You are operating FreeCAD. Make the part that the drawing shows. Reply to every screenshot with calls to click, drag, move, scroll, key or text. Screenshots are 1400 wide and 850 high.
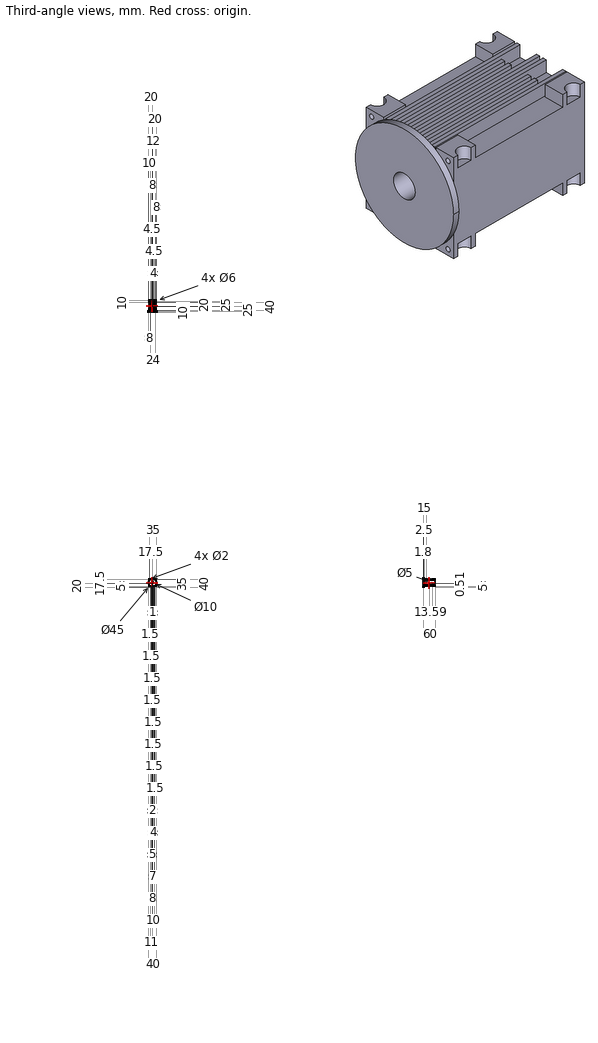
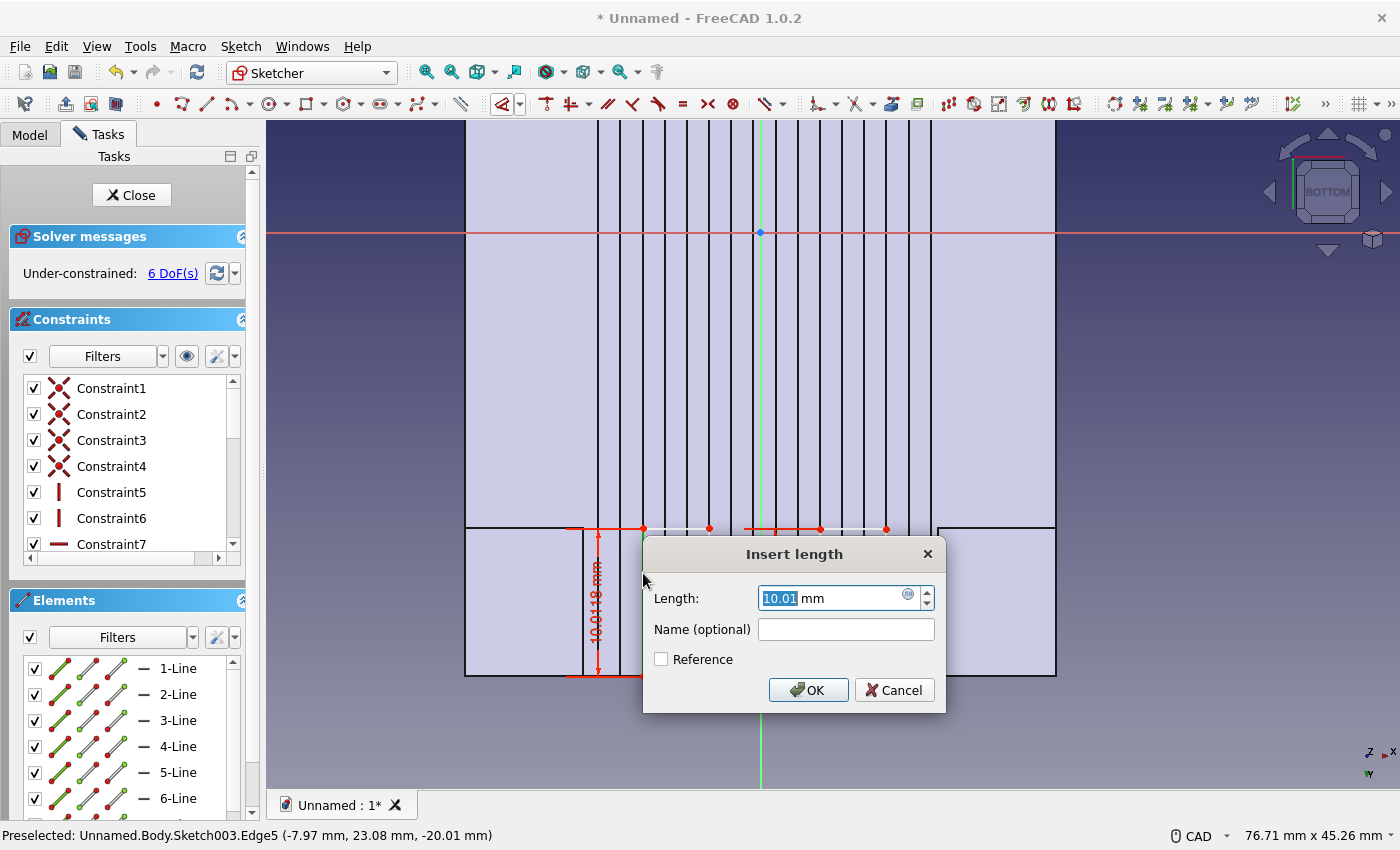
text(10)
key(Return)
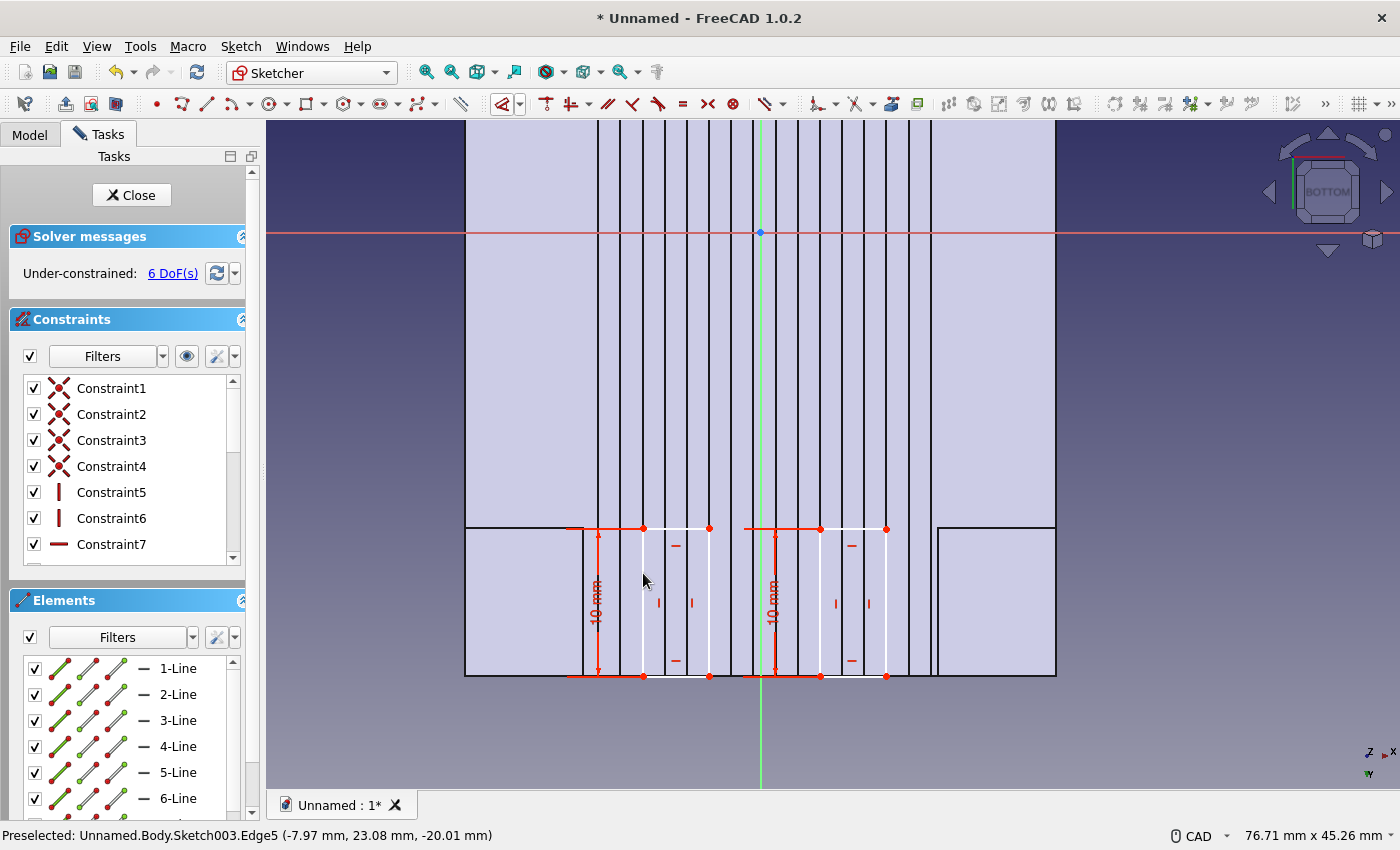
click(820, 529)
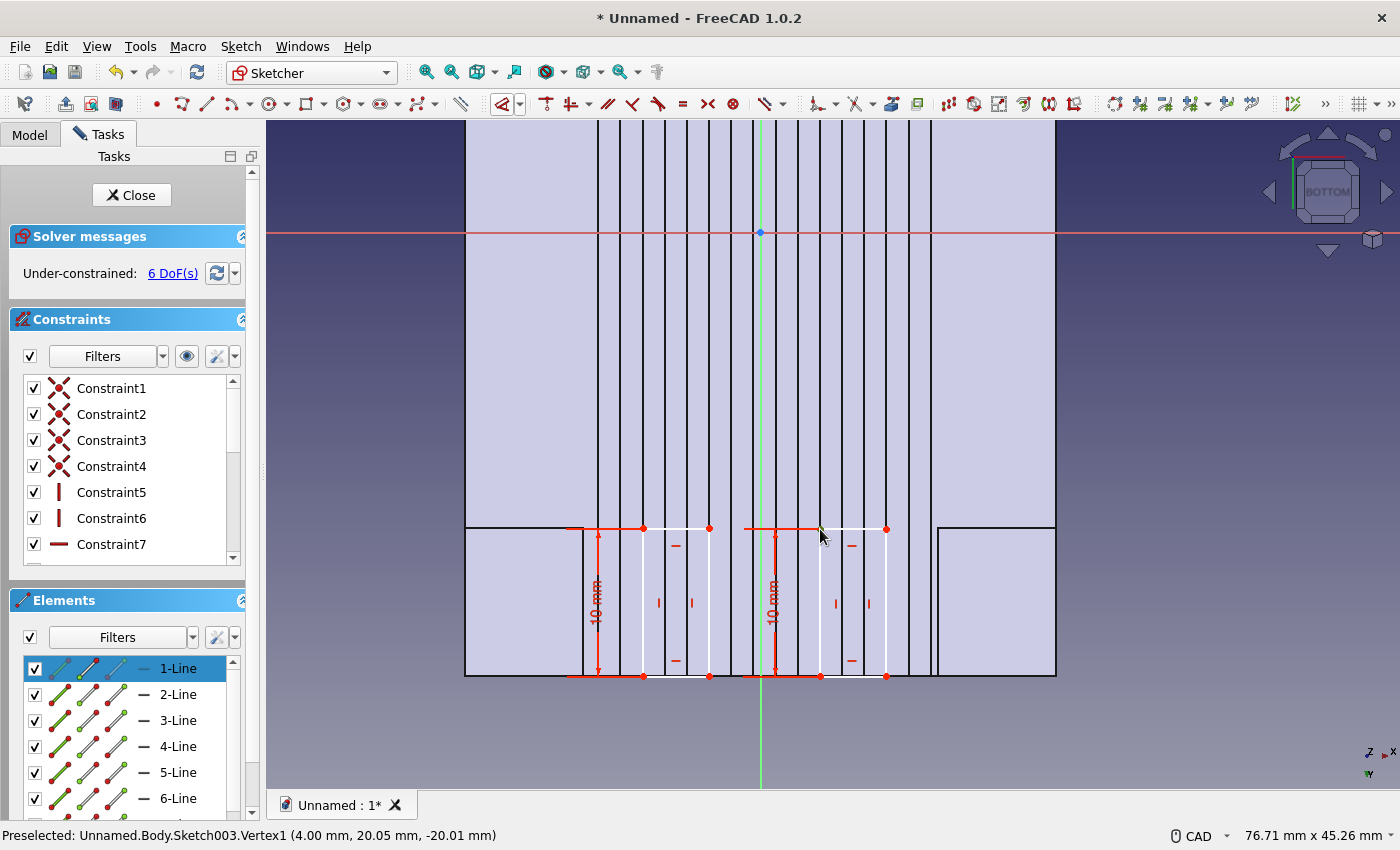
click(520, 104)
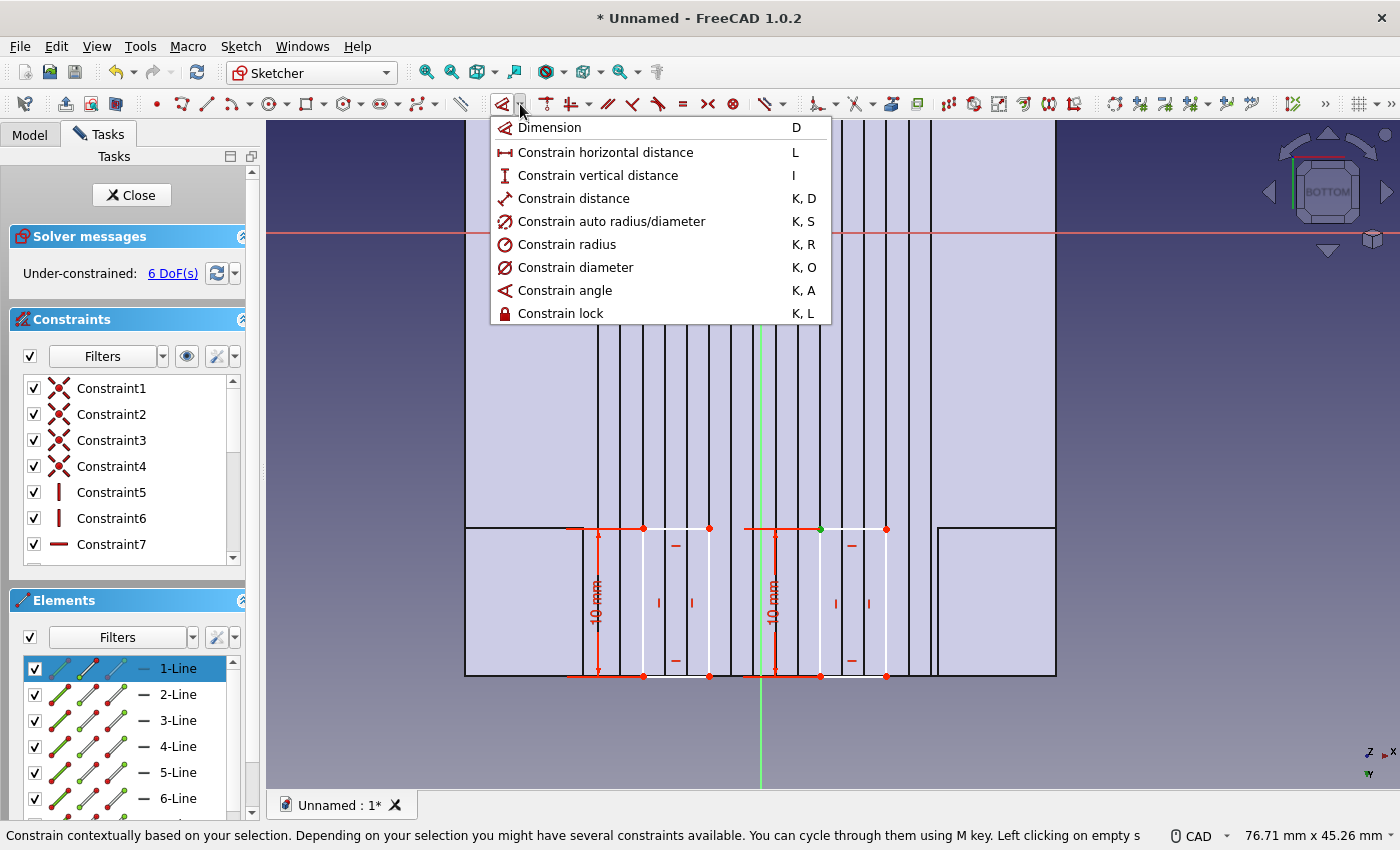
click(661, 152)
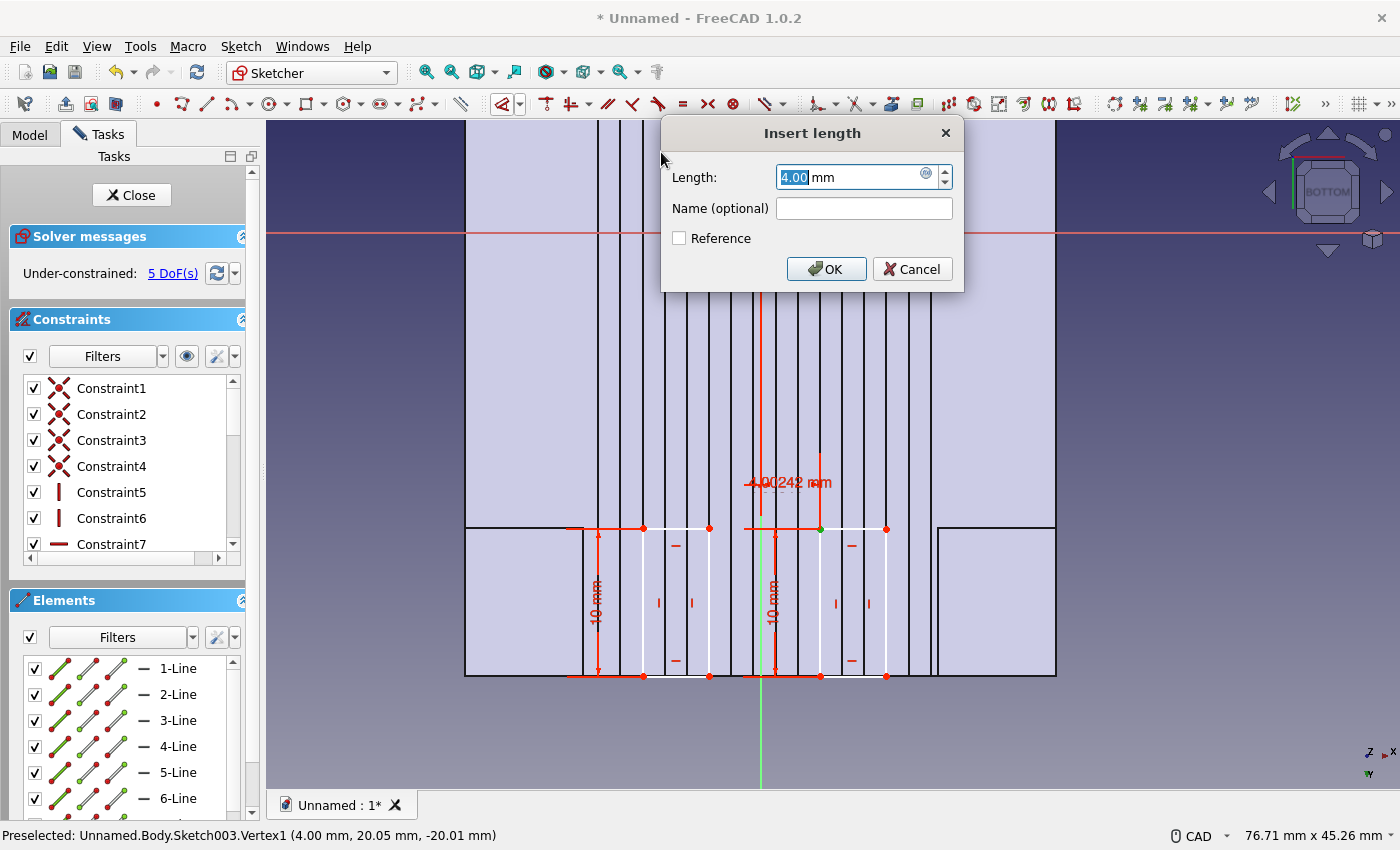
text(4)
key(Return)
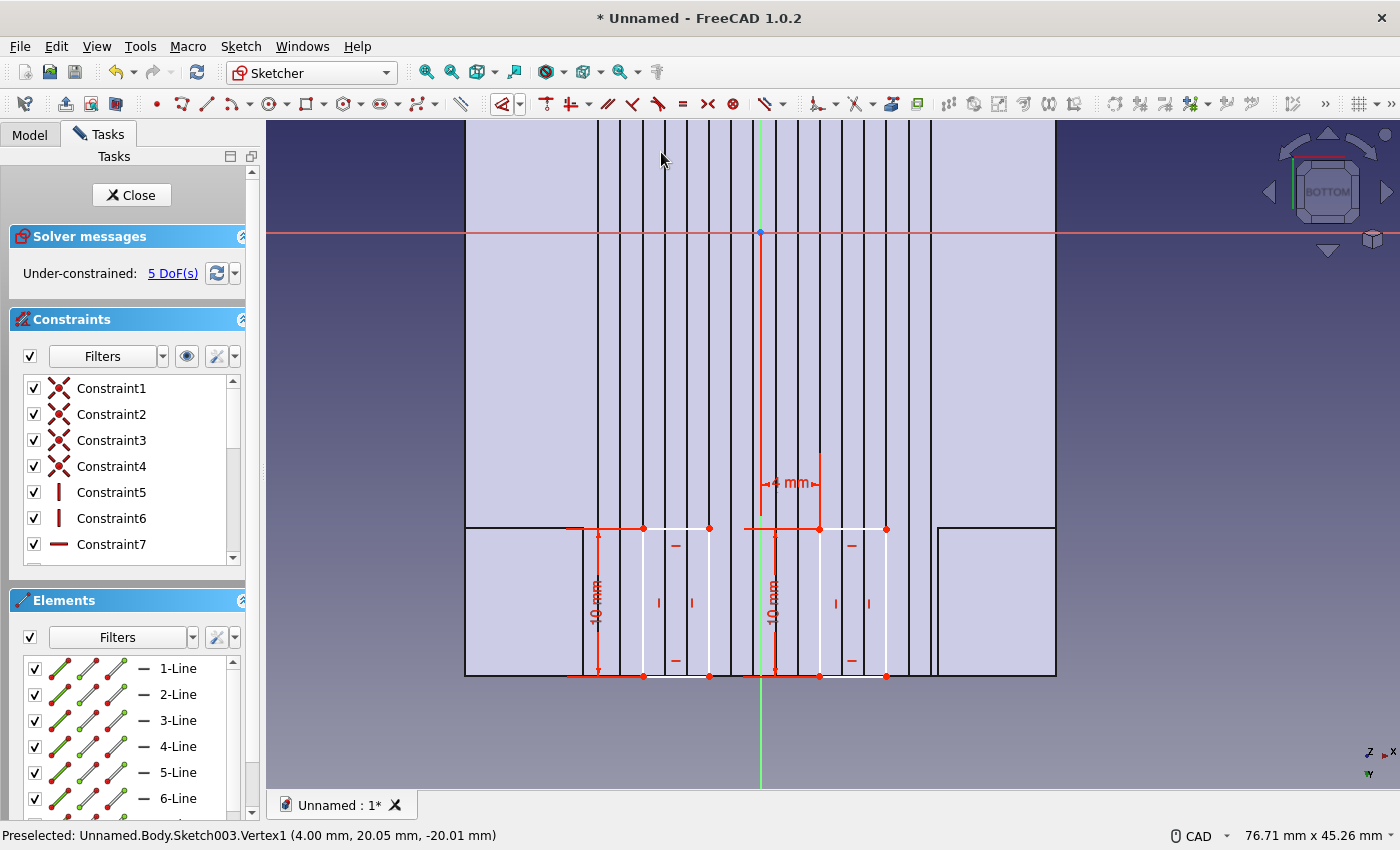
click(643, 529)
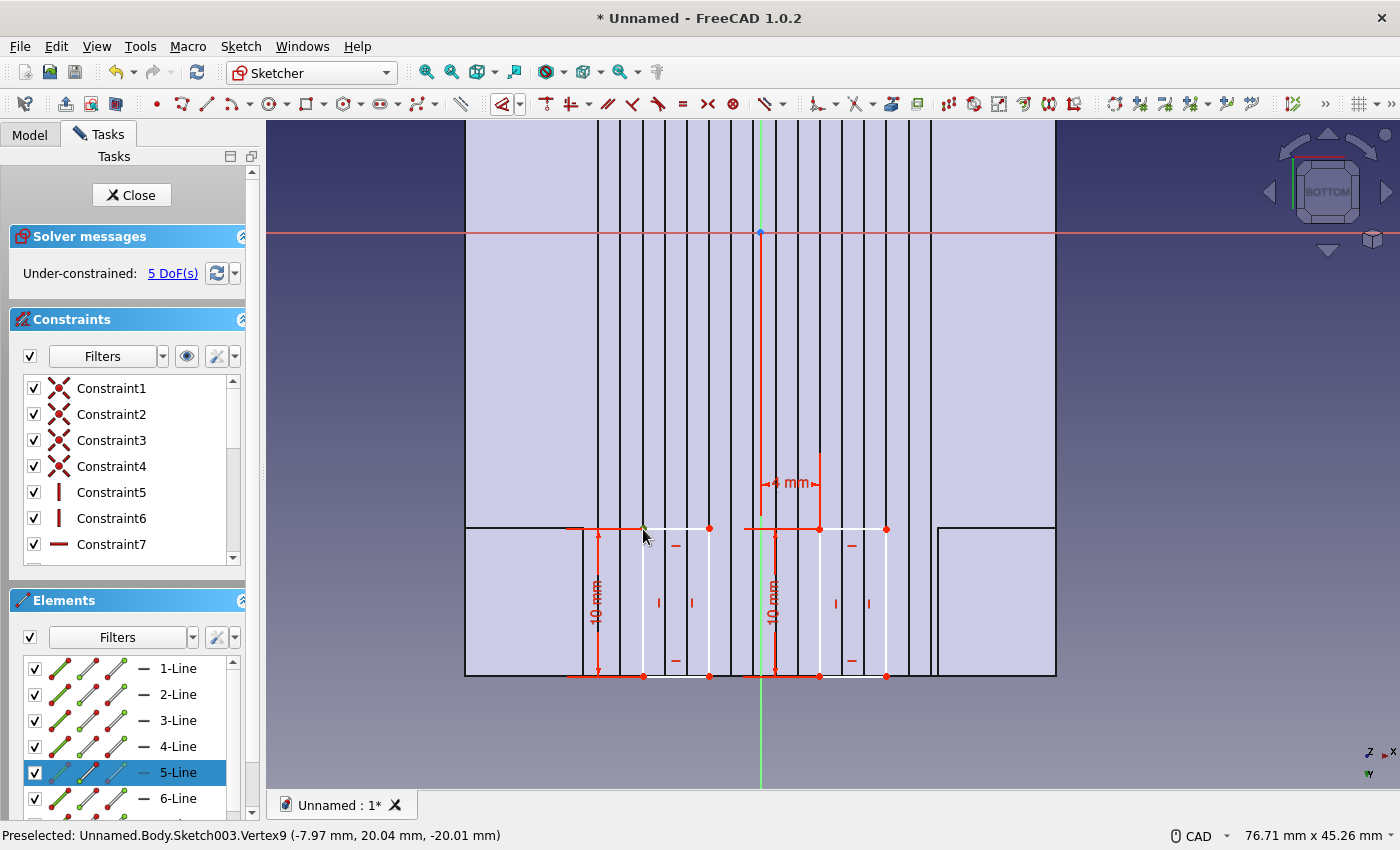
key(l)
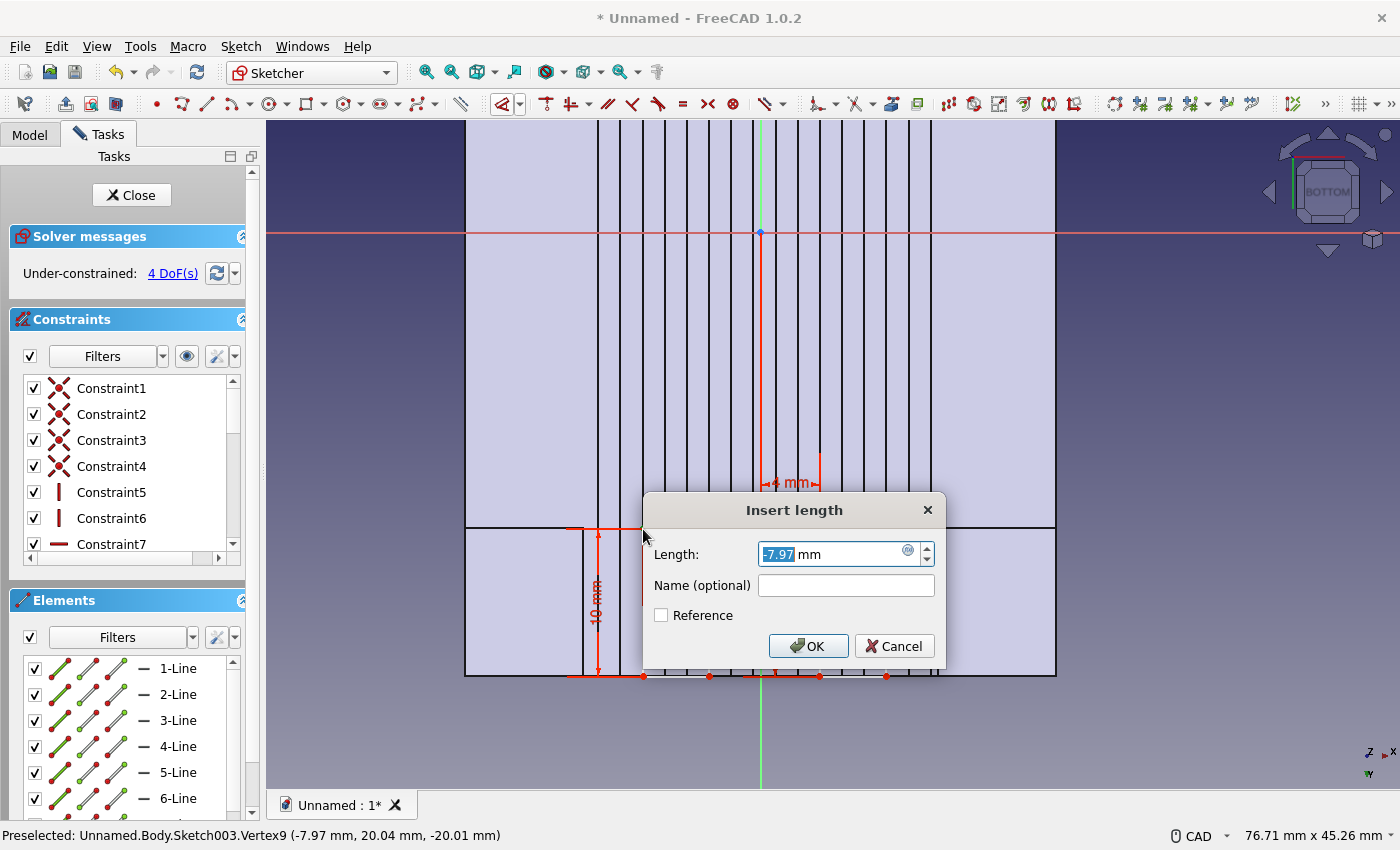
text(-8)
key(Return)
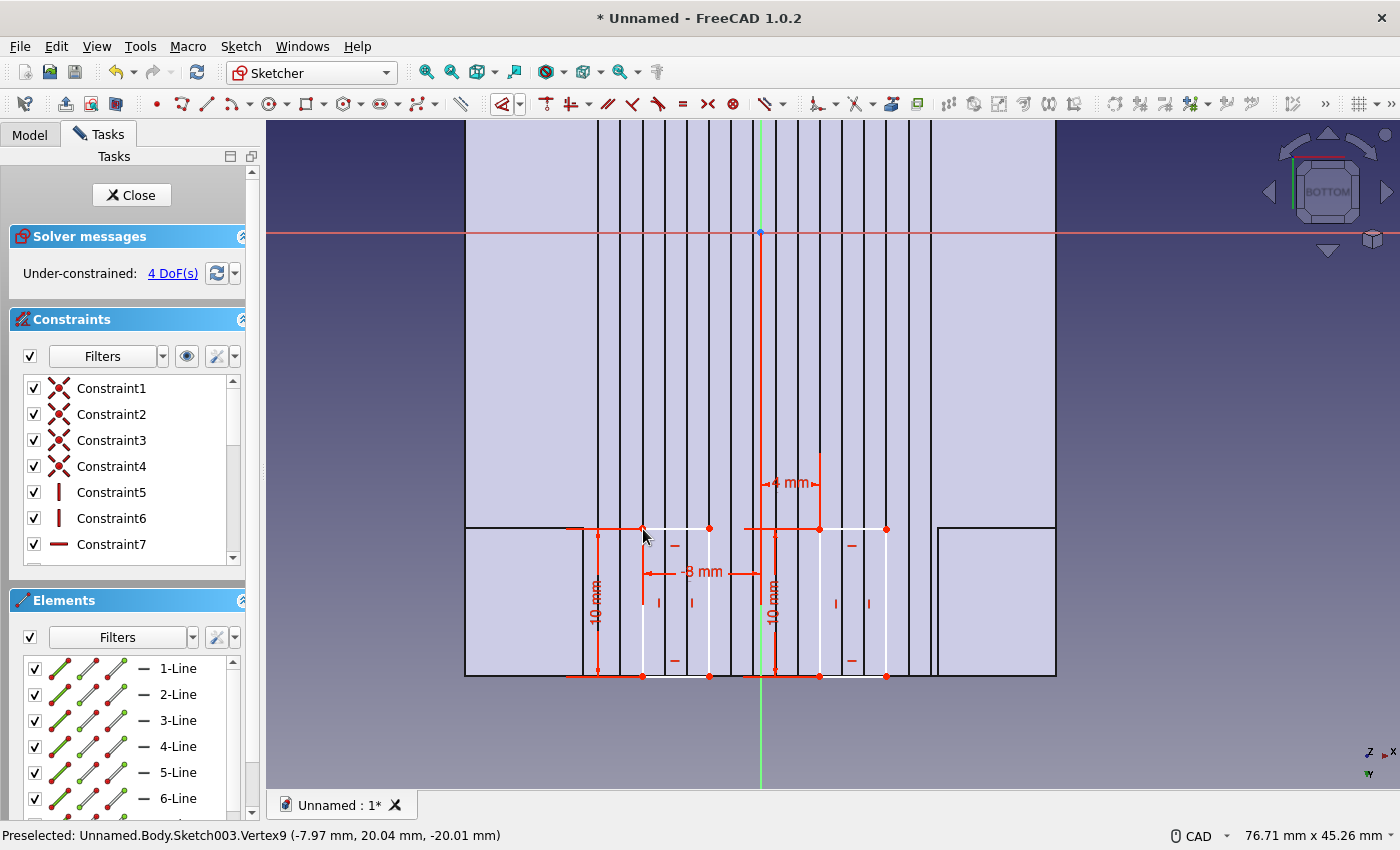
click(840, 677)